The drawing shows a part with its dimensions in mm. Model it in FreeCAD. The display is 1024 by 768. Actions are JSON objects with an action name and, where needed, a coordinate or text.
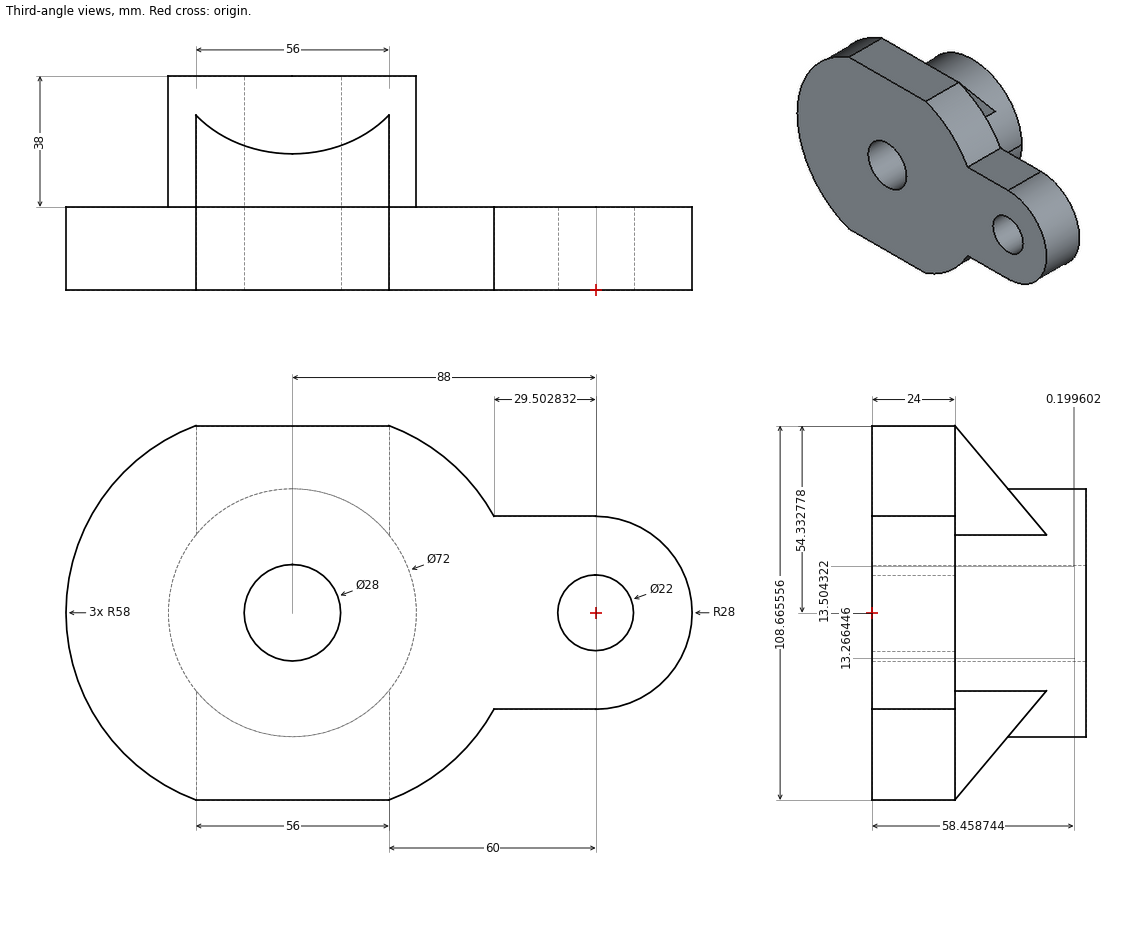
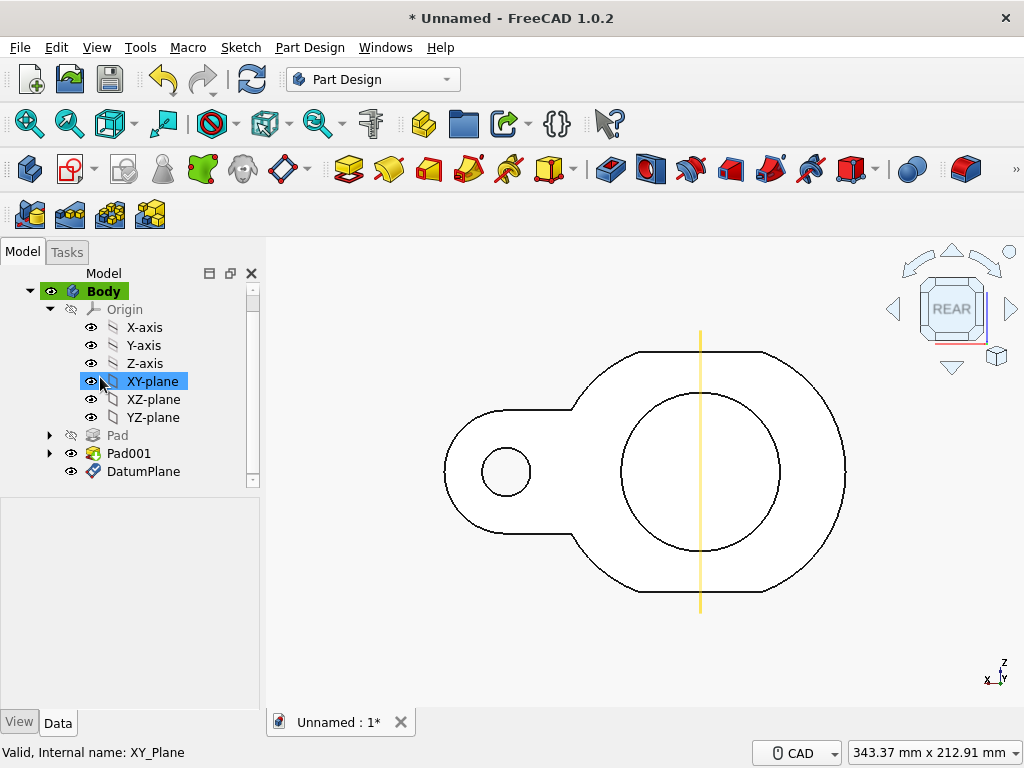
{"action": "left_click", "coordinate": [116, 471]}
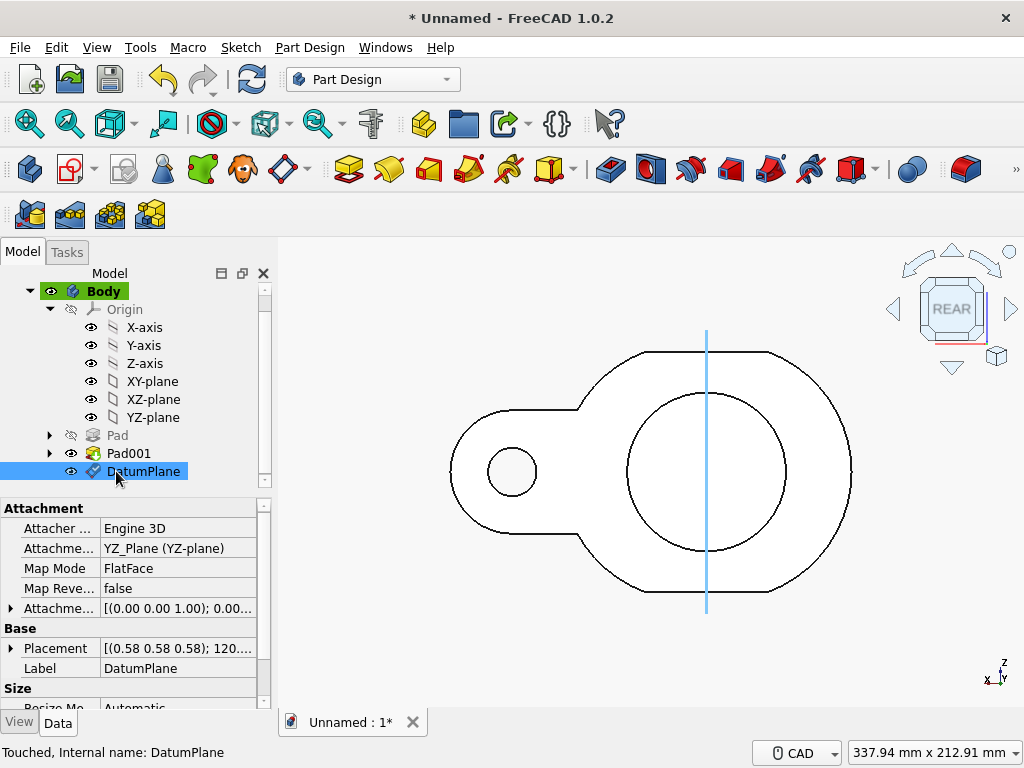
{"action": "left_click", "coordinate": [70, 170]}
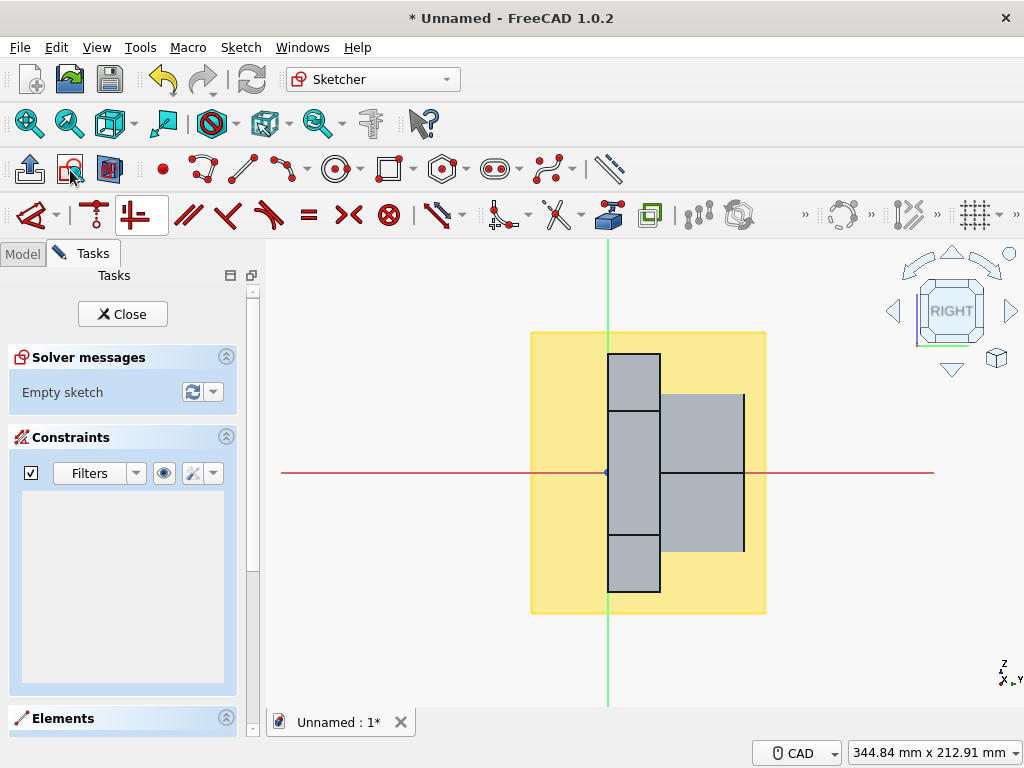
{"action": "left_click", "coordinate": [110, 170]}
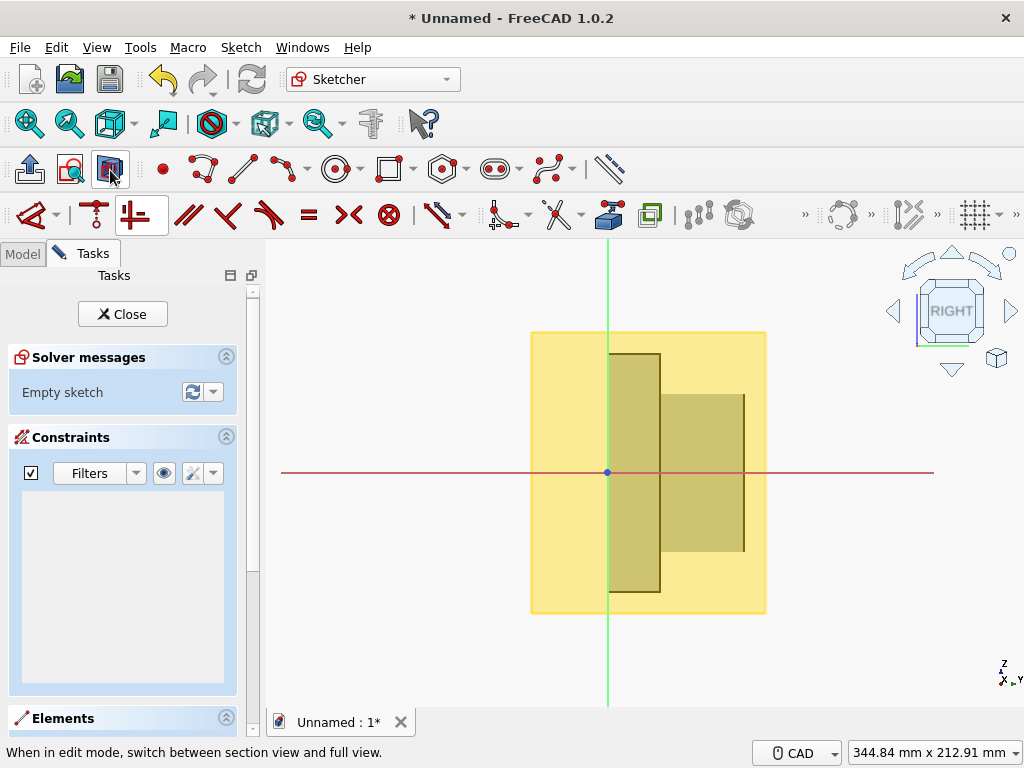
{"action": "left_click", "coordinate": [204, 170]}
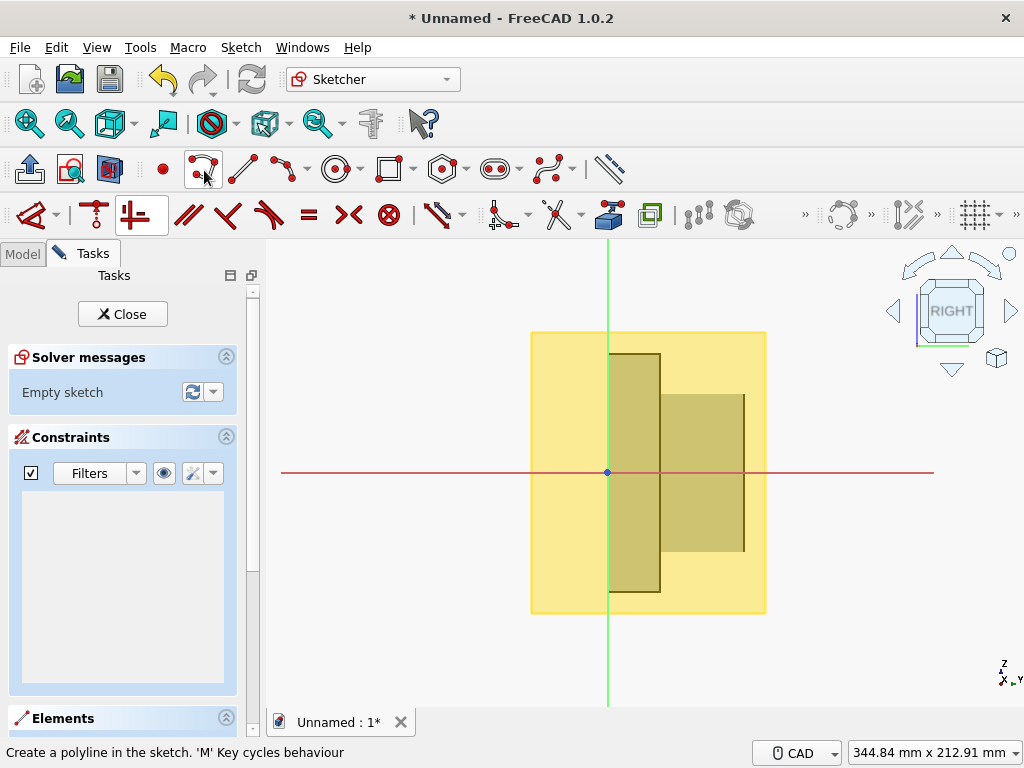
{"action": "left_click", "coordinate": [660, 354]}
{"action": "left_click", "coordinate": [660, 592]}
{"action": "left_click", "coordinate": [736, 502]}
{"action": "left_click", "coordinate": [732, 443]}
{"action": "left_click", "coordinate": [660, 355]}
{"action": "key", "text": "Escape"}
{"action": "key", "text": "Escape"}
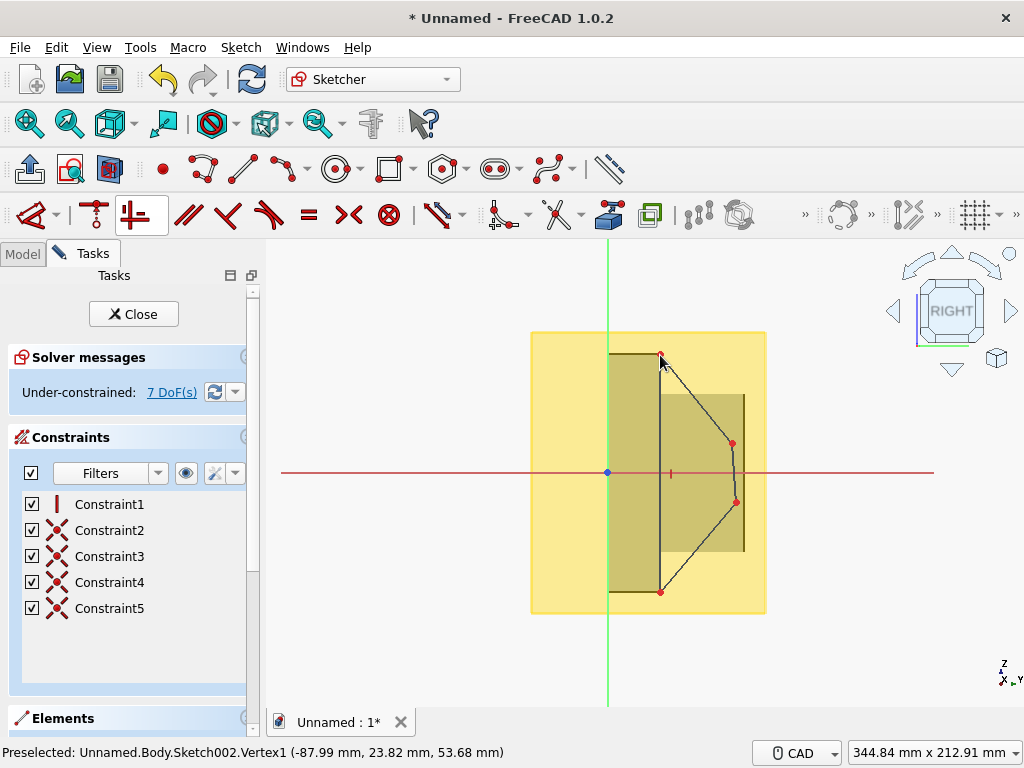
{"action": "left_click", "coordinate": [32, 216]}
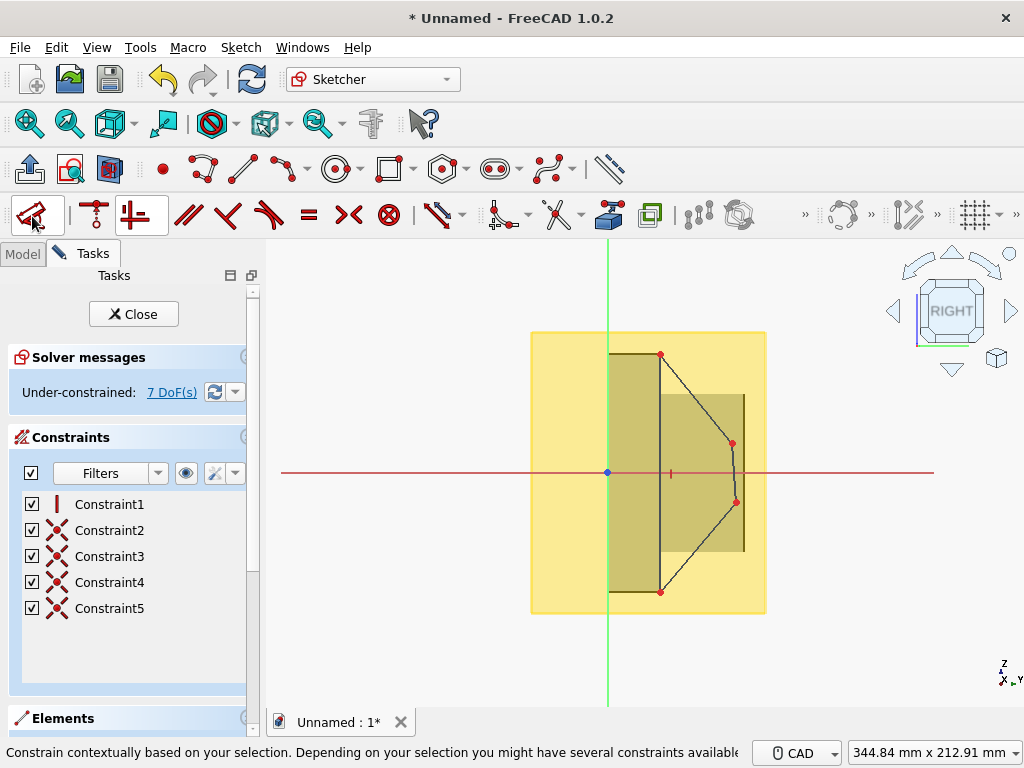
{"action": "left_click", "coordinate": [660, 355]}
{"action": "left_click", "coordinate": [634, 321]}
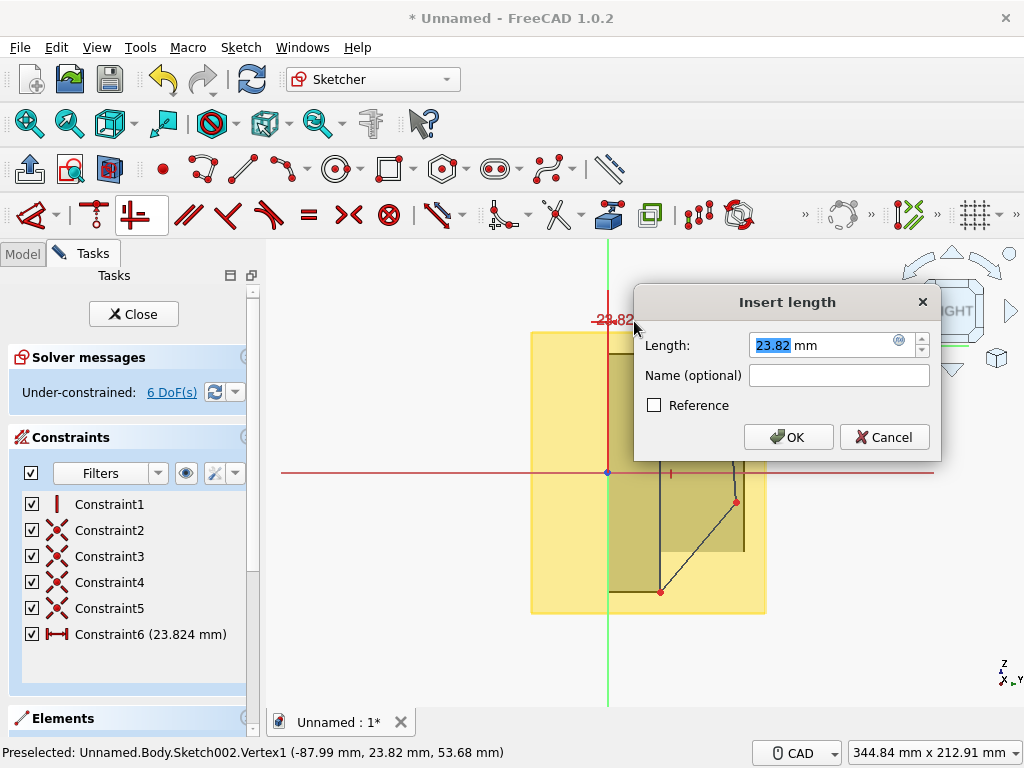
{"action": "type", "text": "24"}
{"action": "key", "text": "Return"}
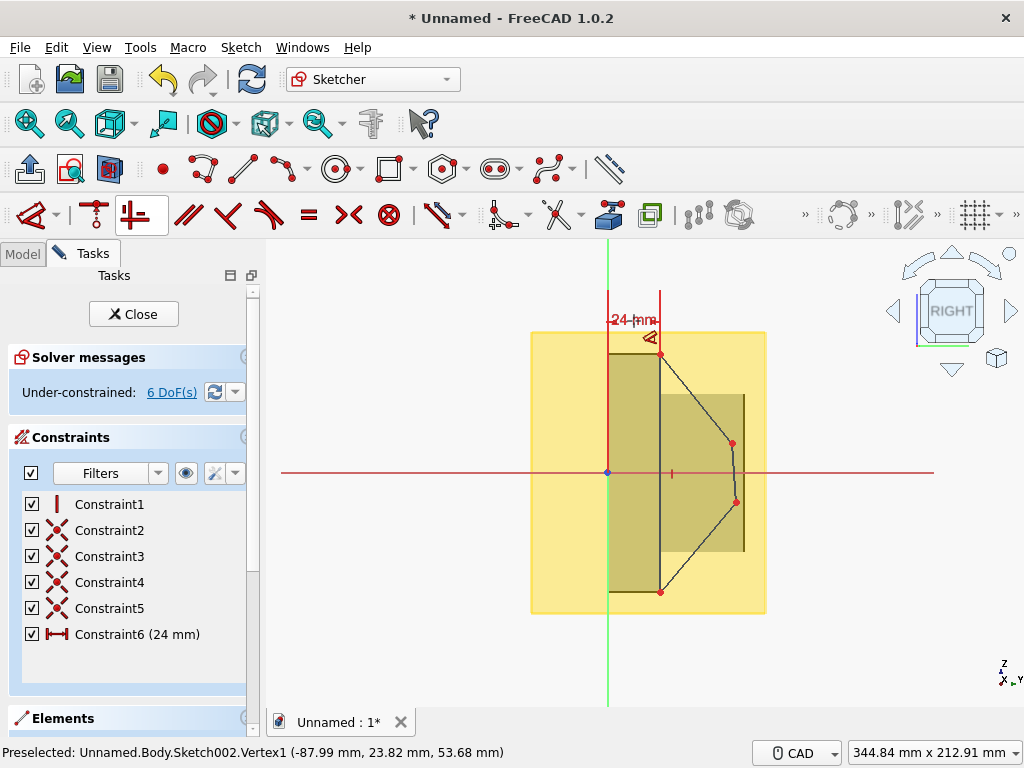
{"action": "scroll", "coordinate": [735, 485], "scroll_direction": "up", "scroll_amount": 23}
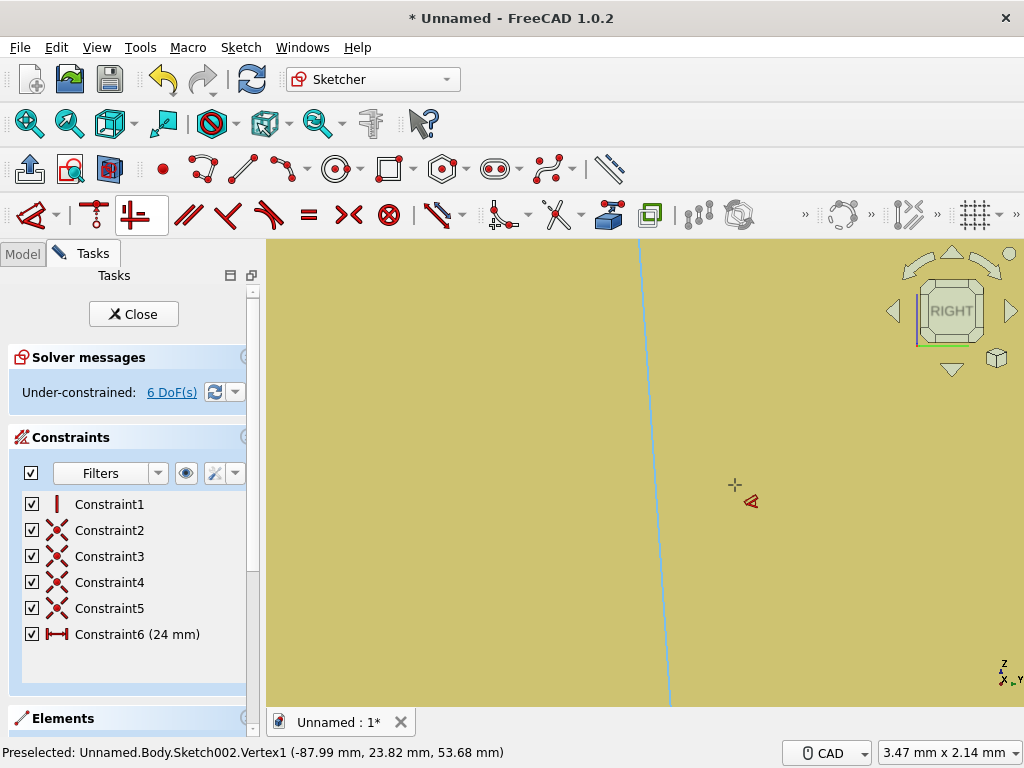
{"action": "left_click", "coordinate": [654, 463]}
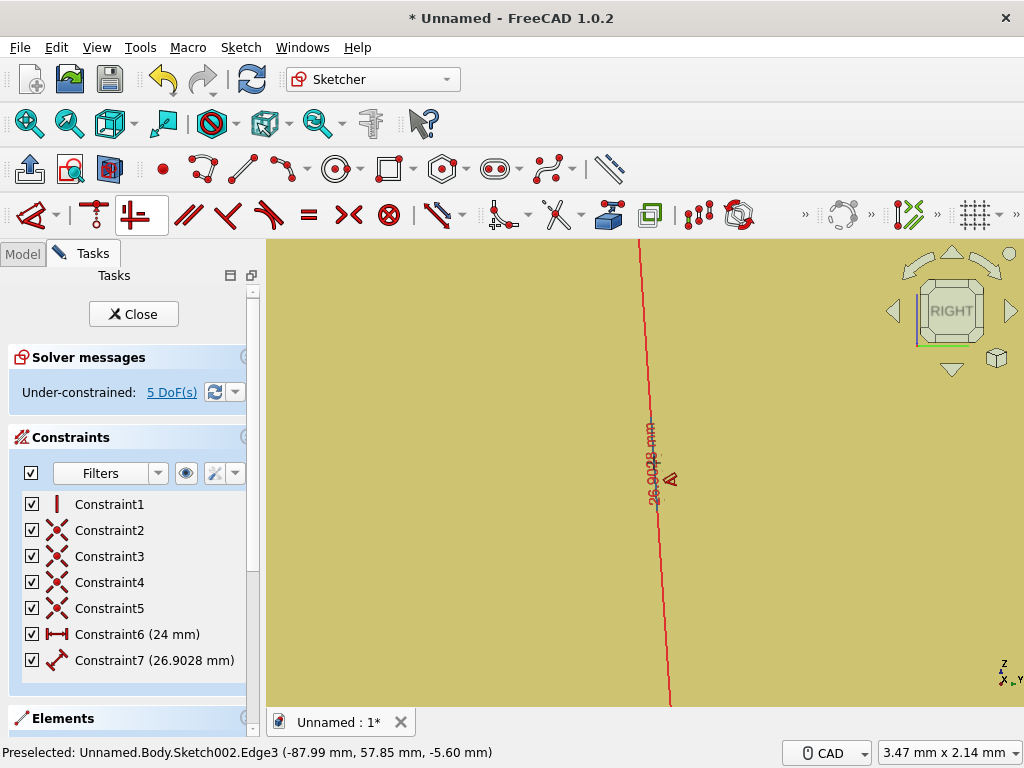
{"action": "key", "text": "Escape"}
{"action": "key", "text": "Escape"}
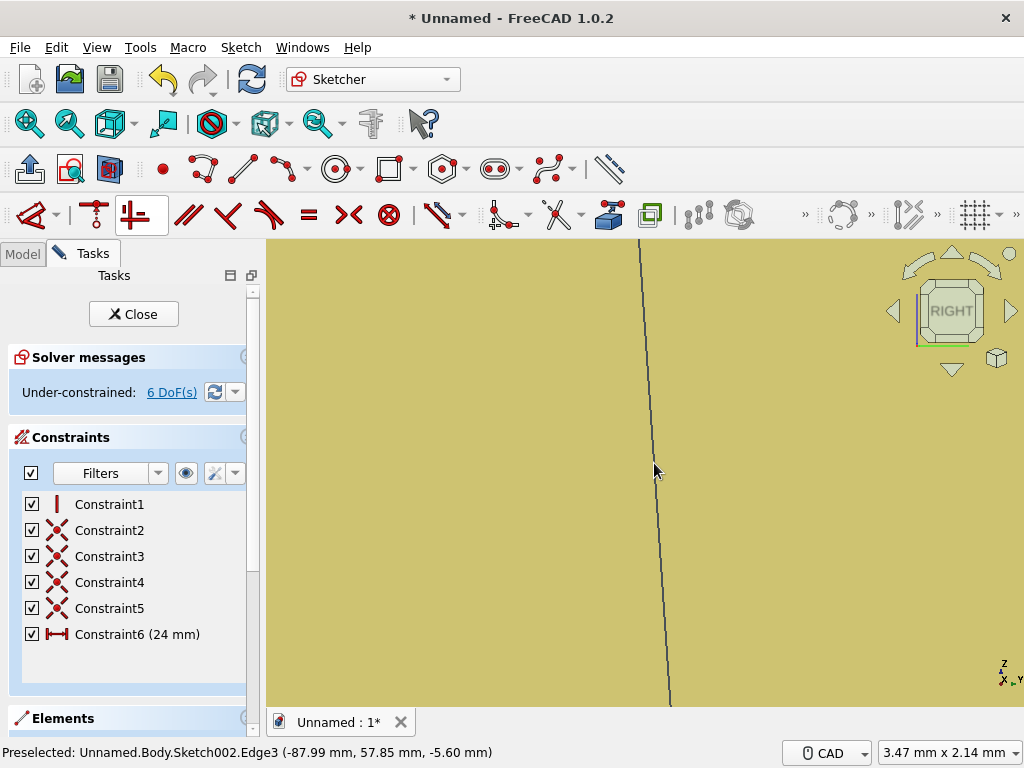
{"action": "left_click", "coordinate": [654, 463]}